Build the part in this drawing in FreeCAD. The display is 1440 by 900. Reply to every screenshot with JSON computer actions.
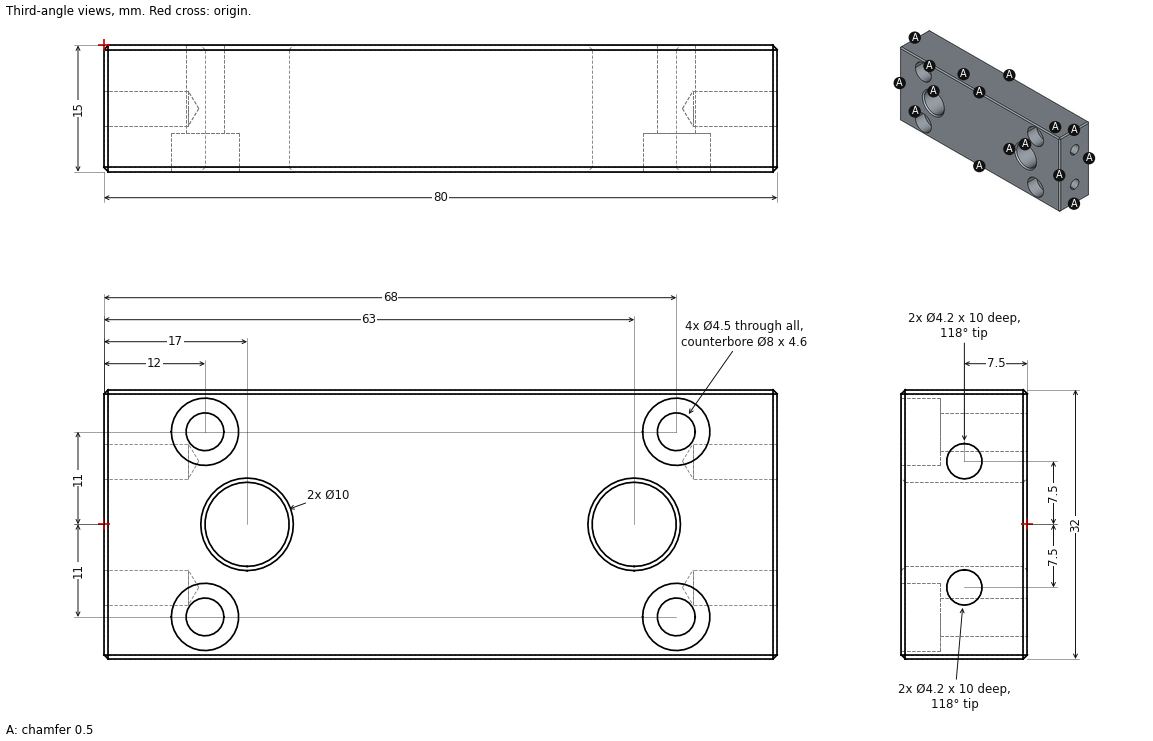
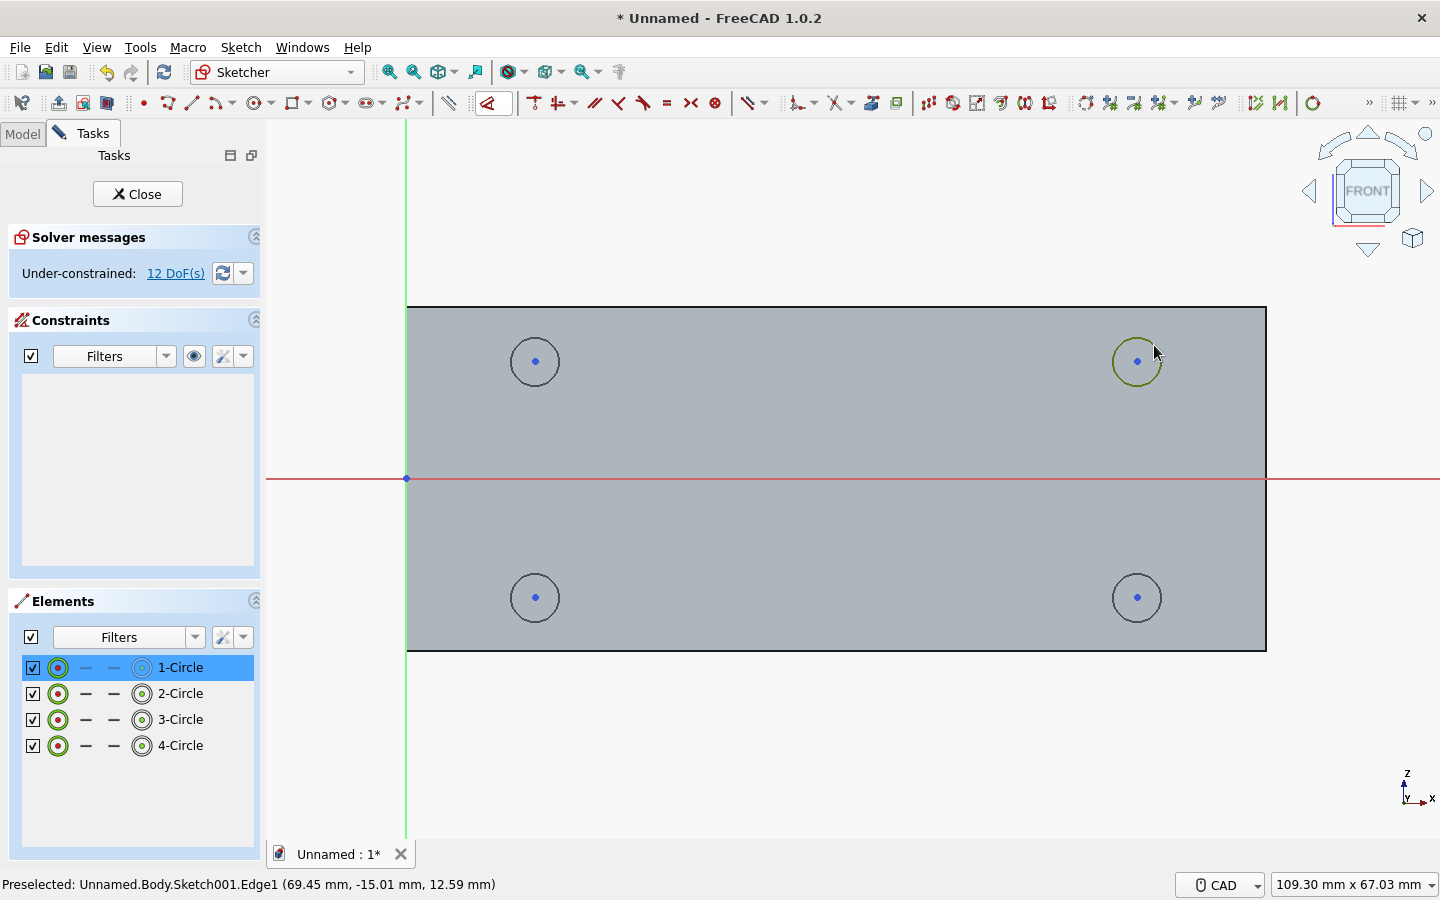
{"action": "left_click", "coordinate": [1154, 581]}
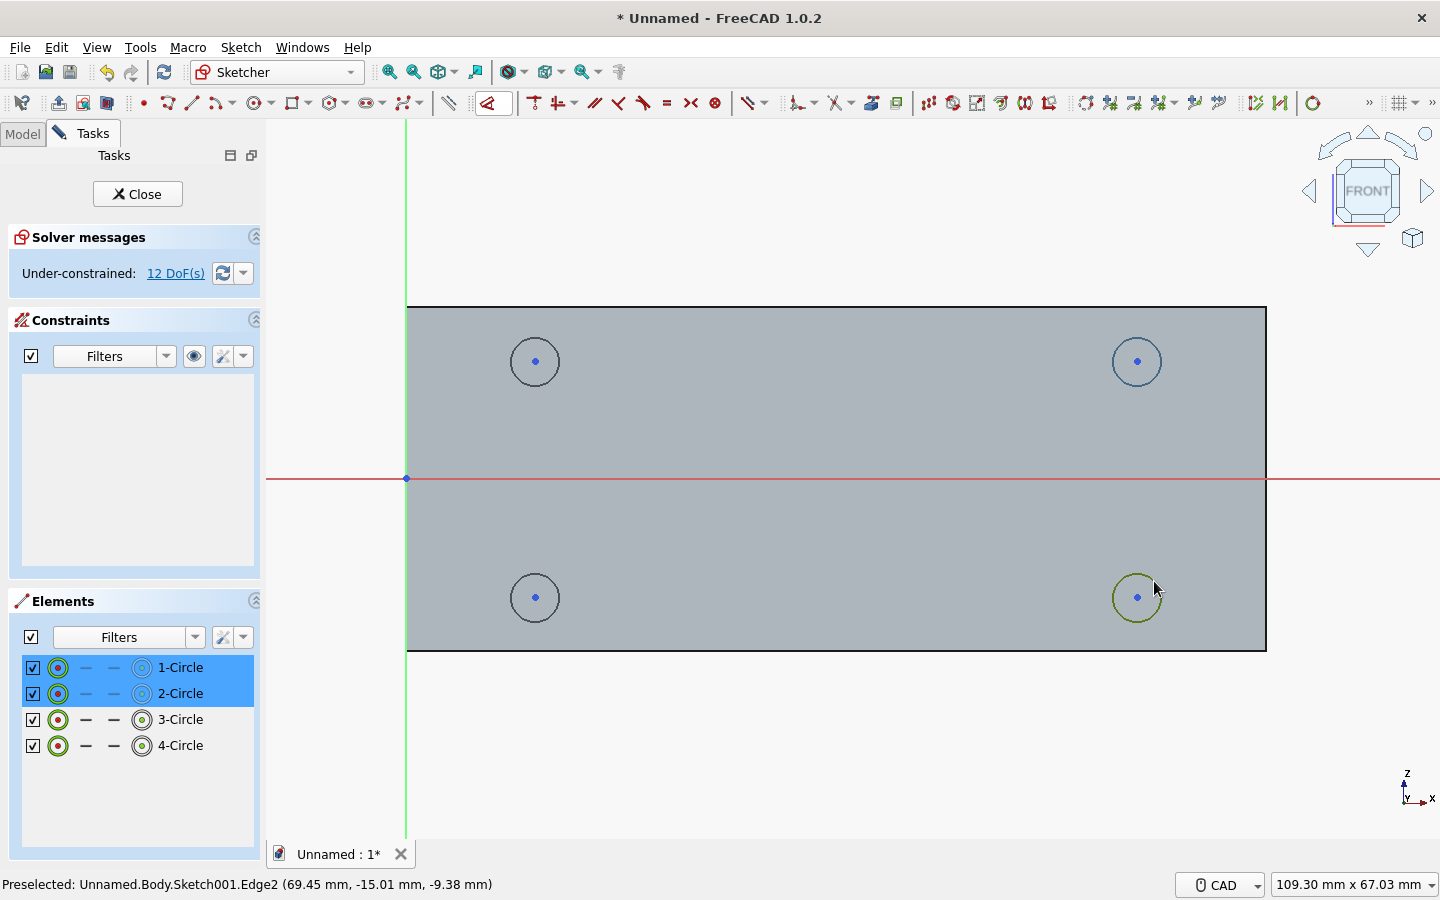
{"action": "left_click", "coordinate": [552, 345]}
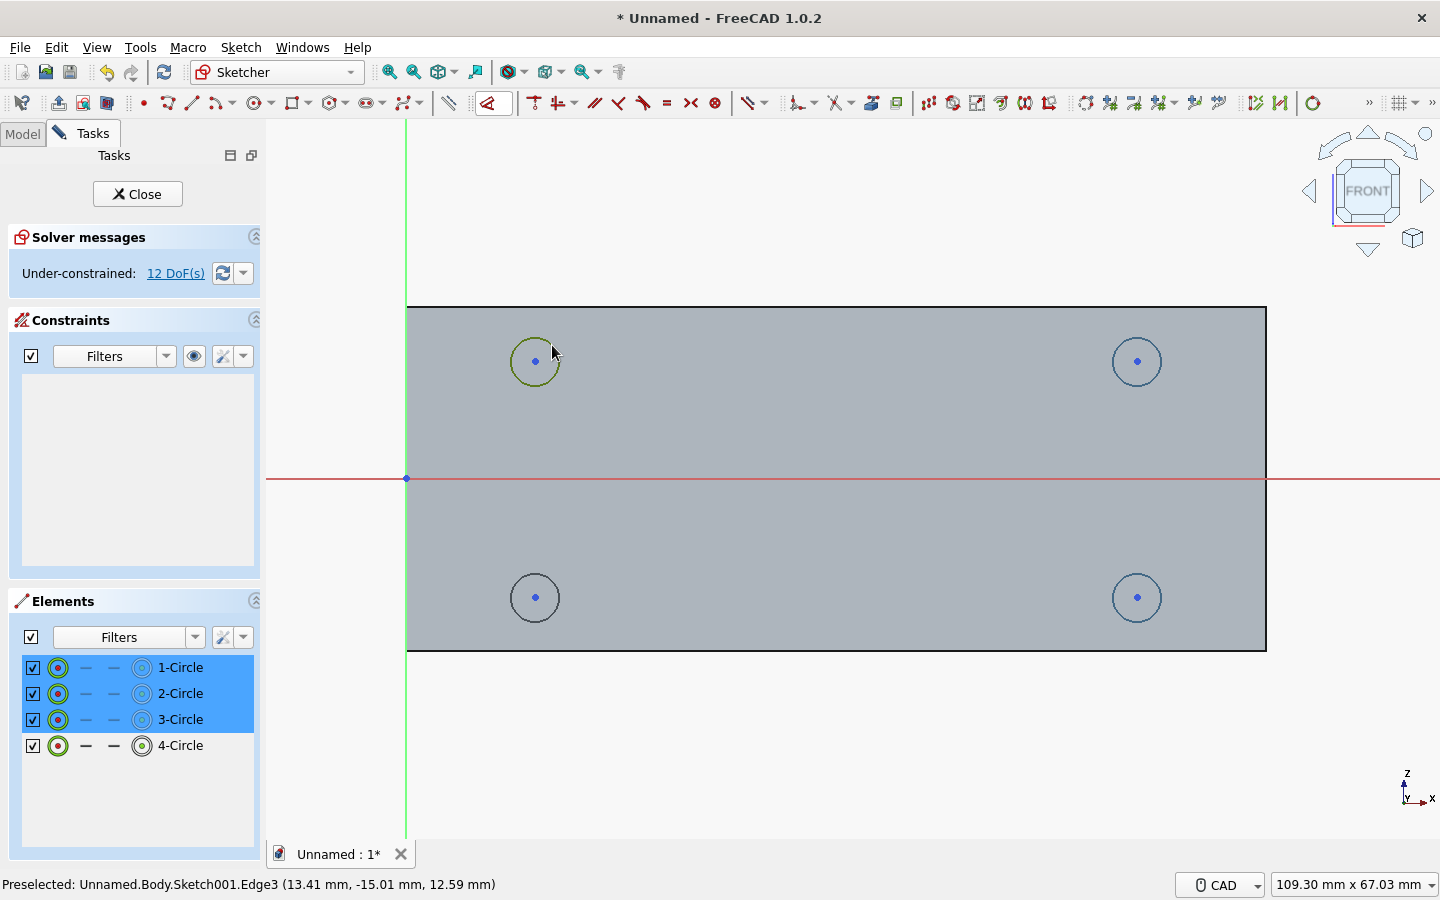
{"action": "left_click", "coordinate": [552, 581]}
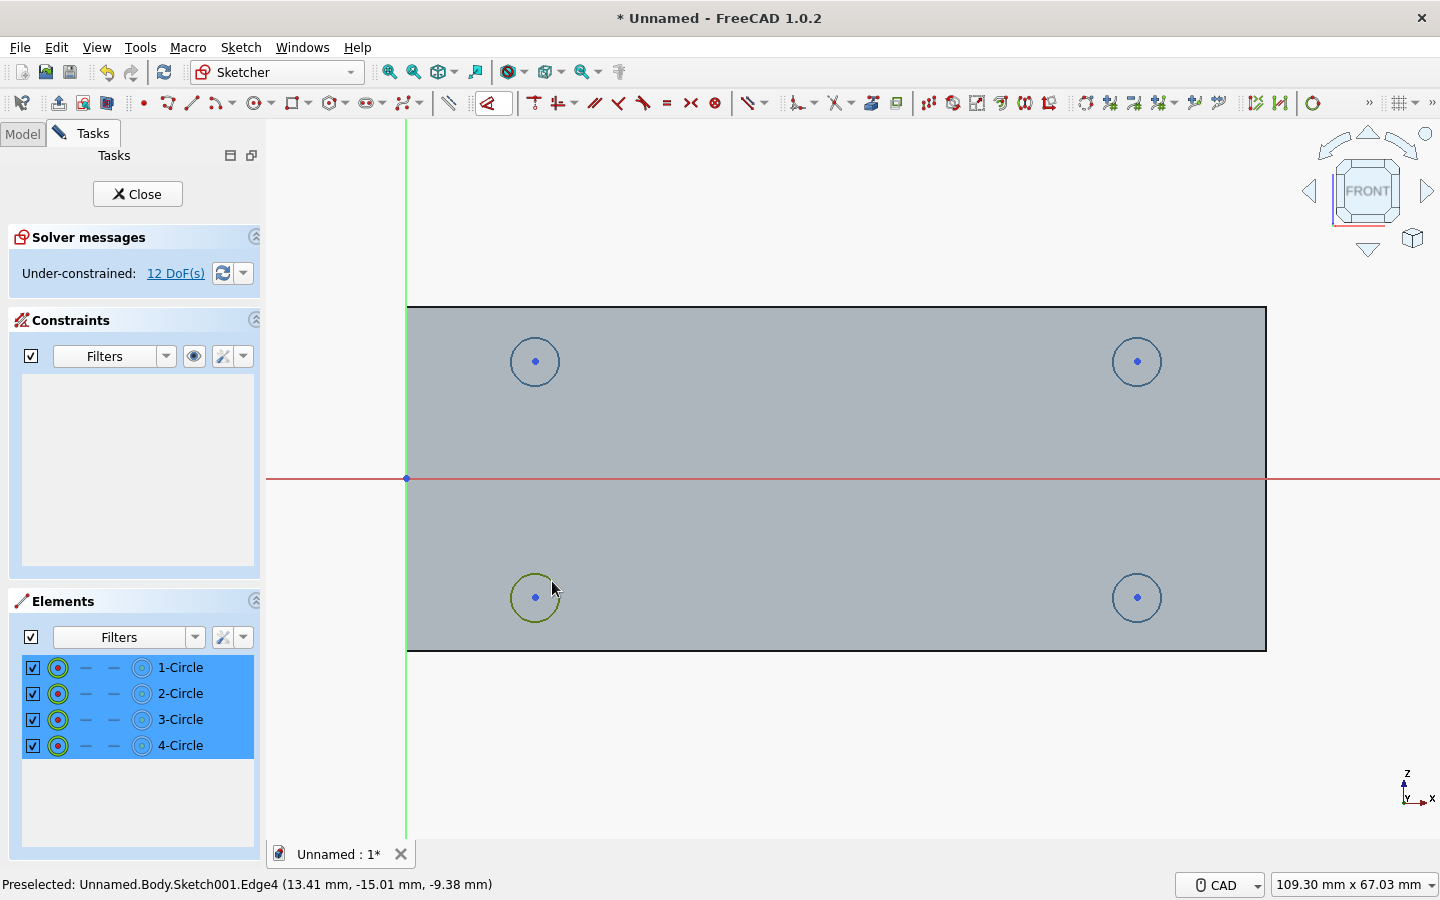
{"action": "left_click", "coordinate": [668, 104]}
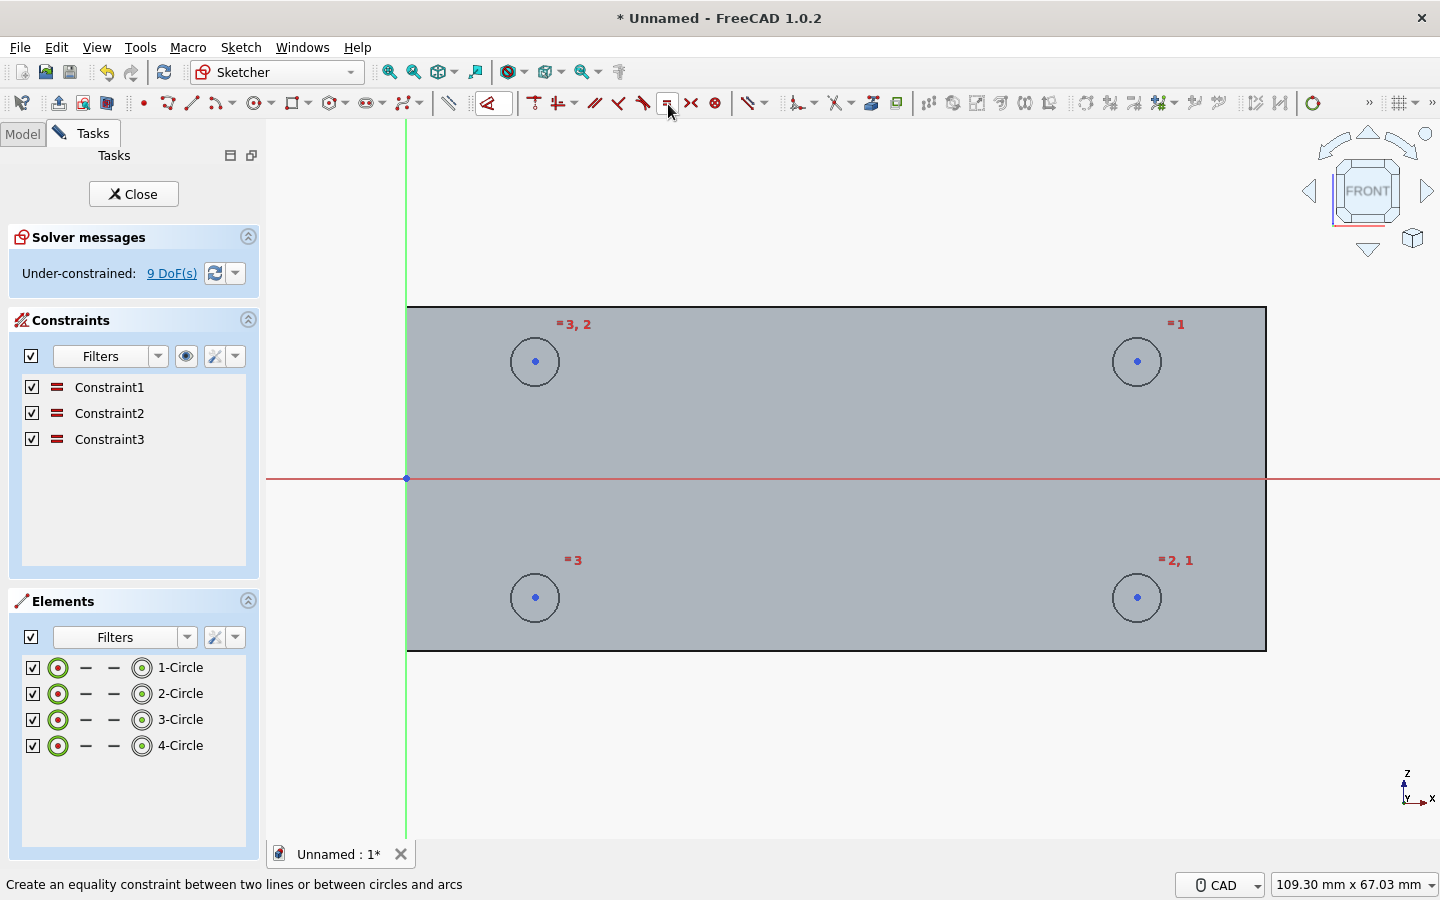
{"action": "left_click", "coordinate": [1154, 345]}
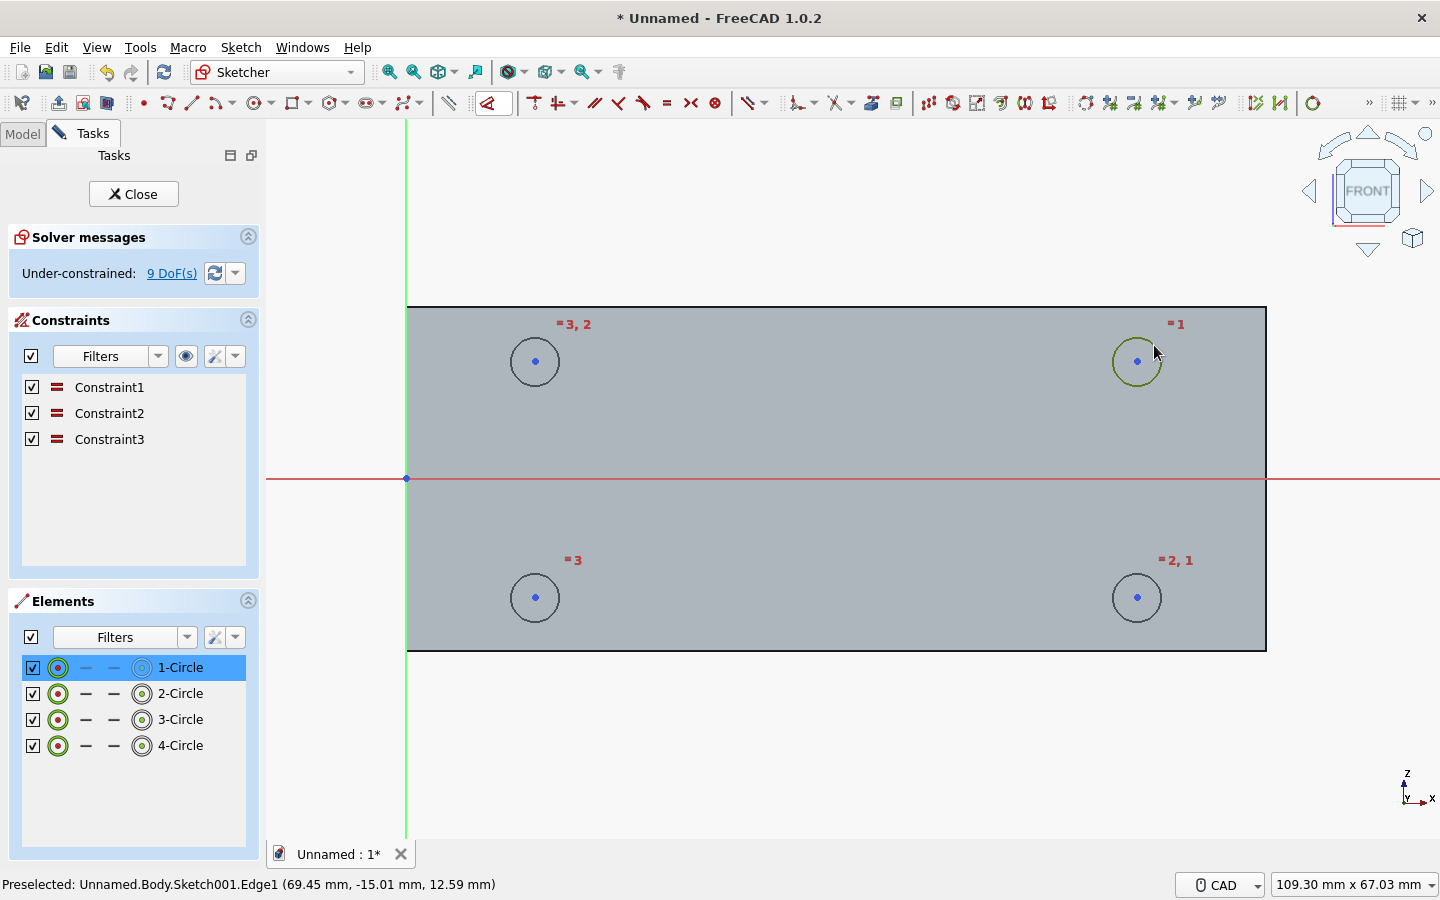
{"action": "left_click", "coordinate": [506, 104]}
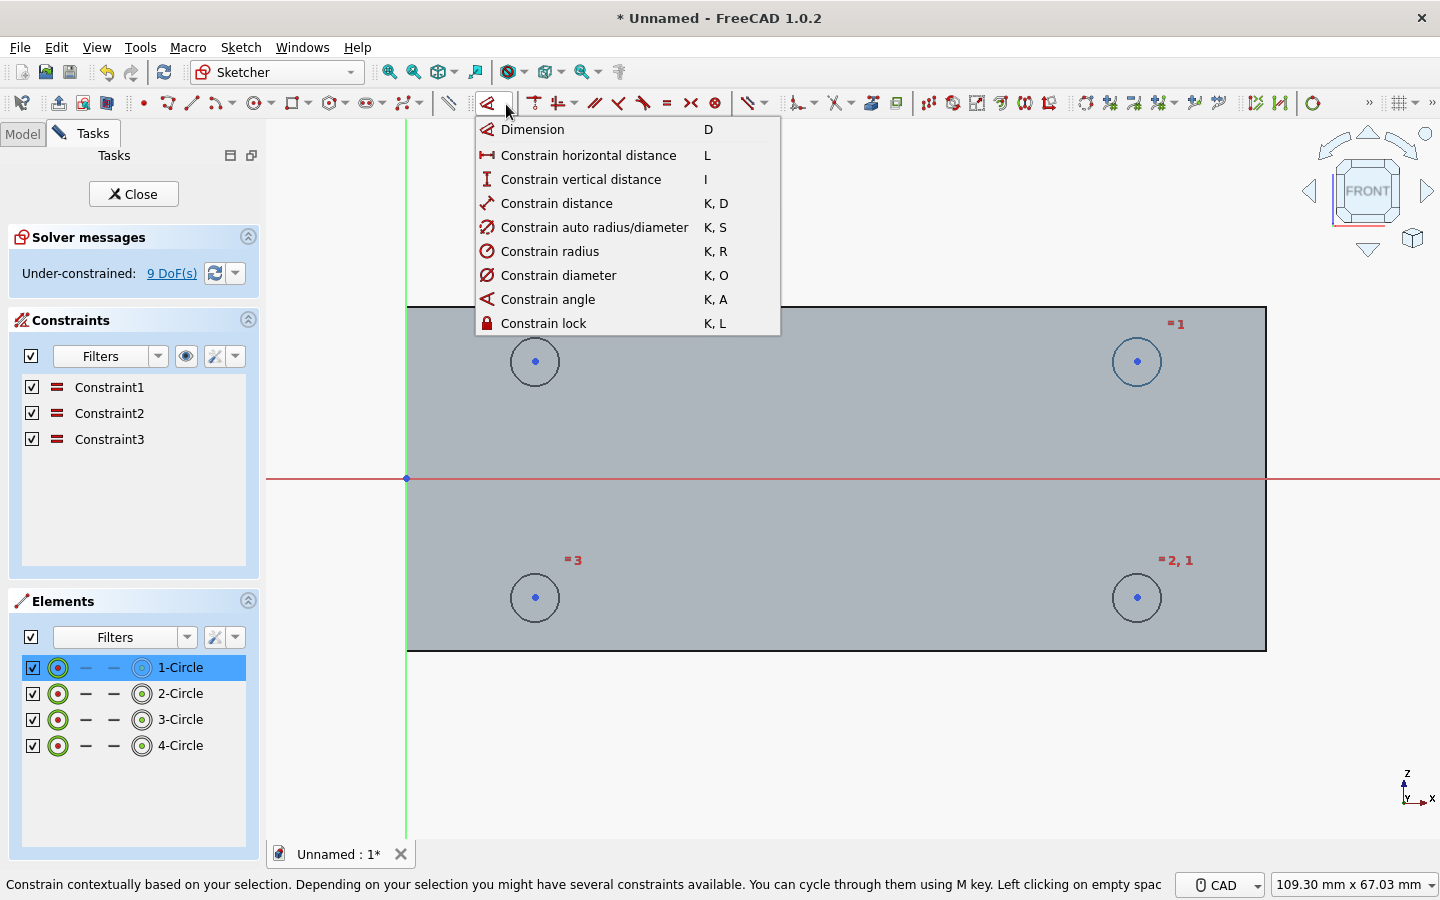
{"action": "left_click", "coordinate": [628, 275]}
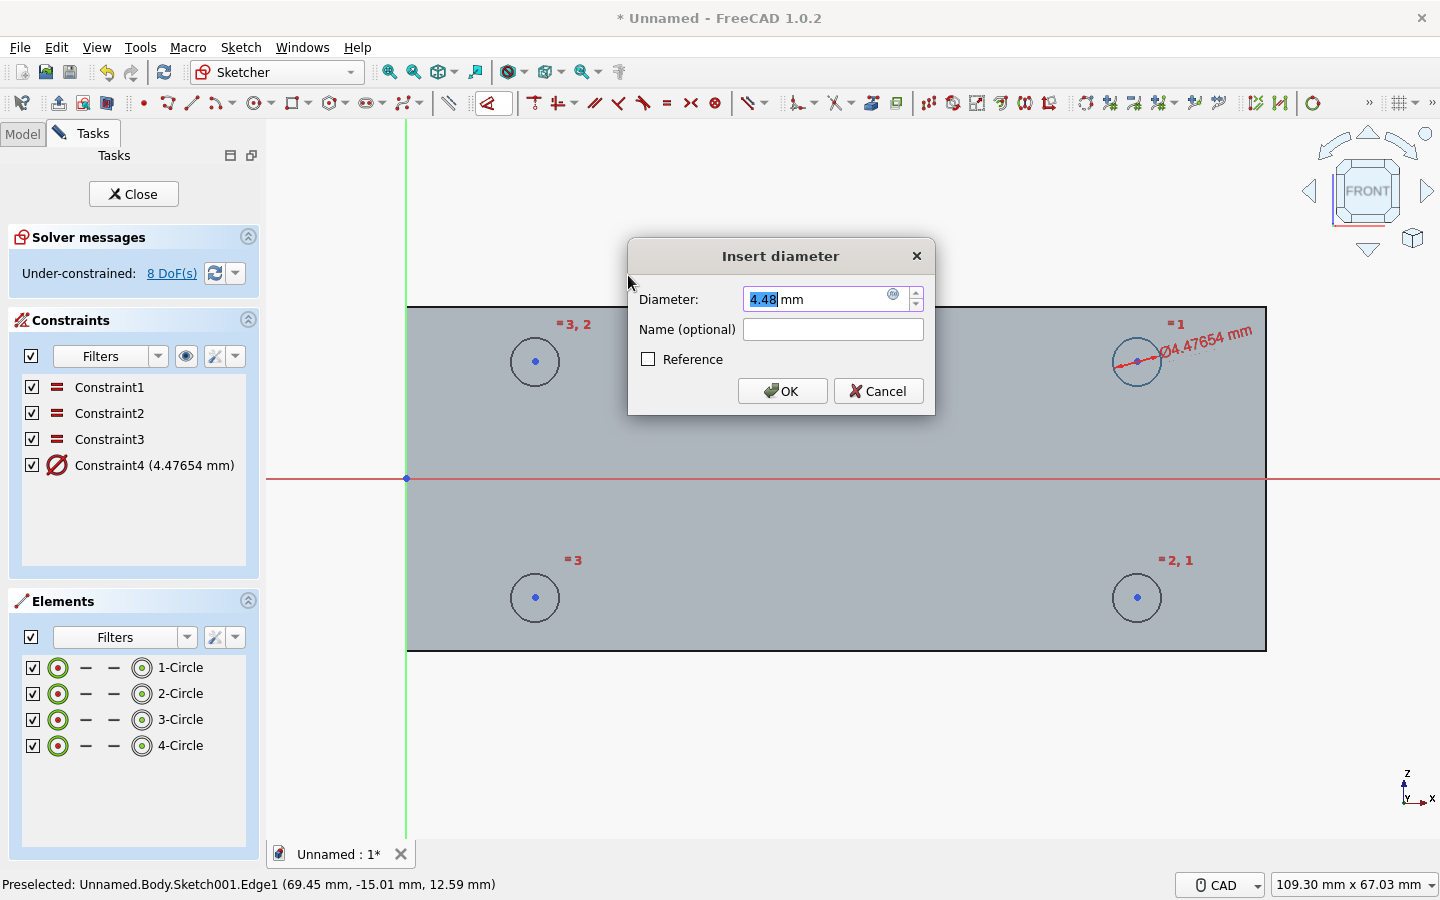
{"action": "type", "text": "4.5"}
{"action": "key", "text": "Return"}